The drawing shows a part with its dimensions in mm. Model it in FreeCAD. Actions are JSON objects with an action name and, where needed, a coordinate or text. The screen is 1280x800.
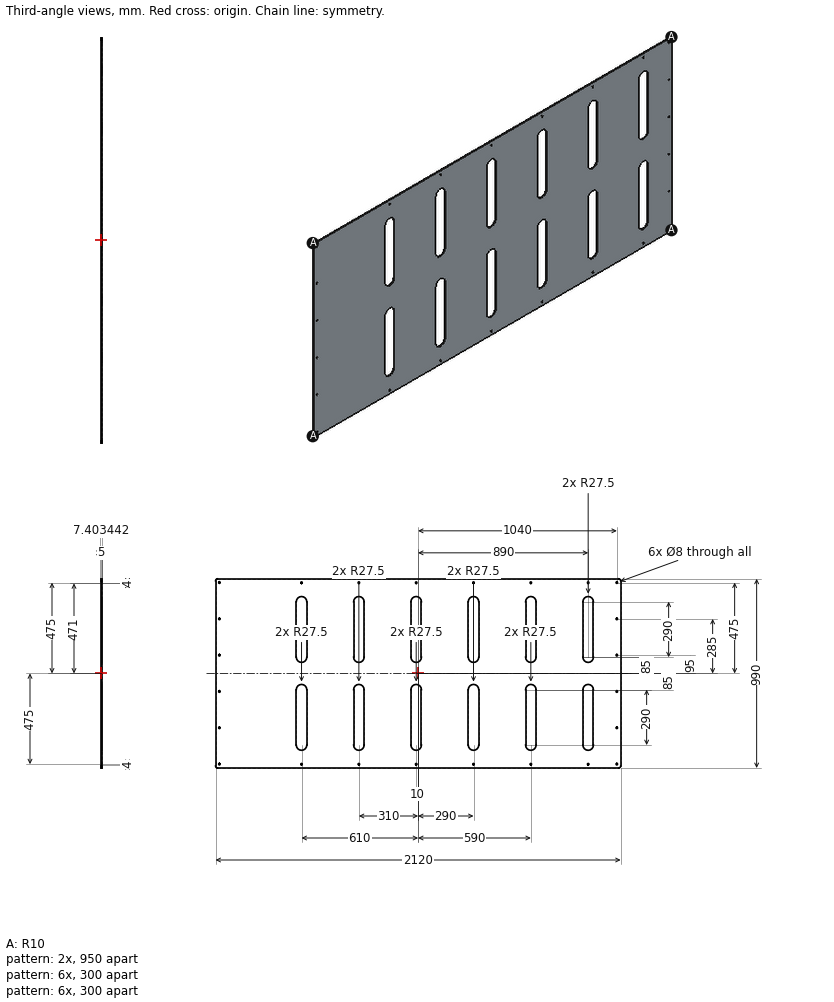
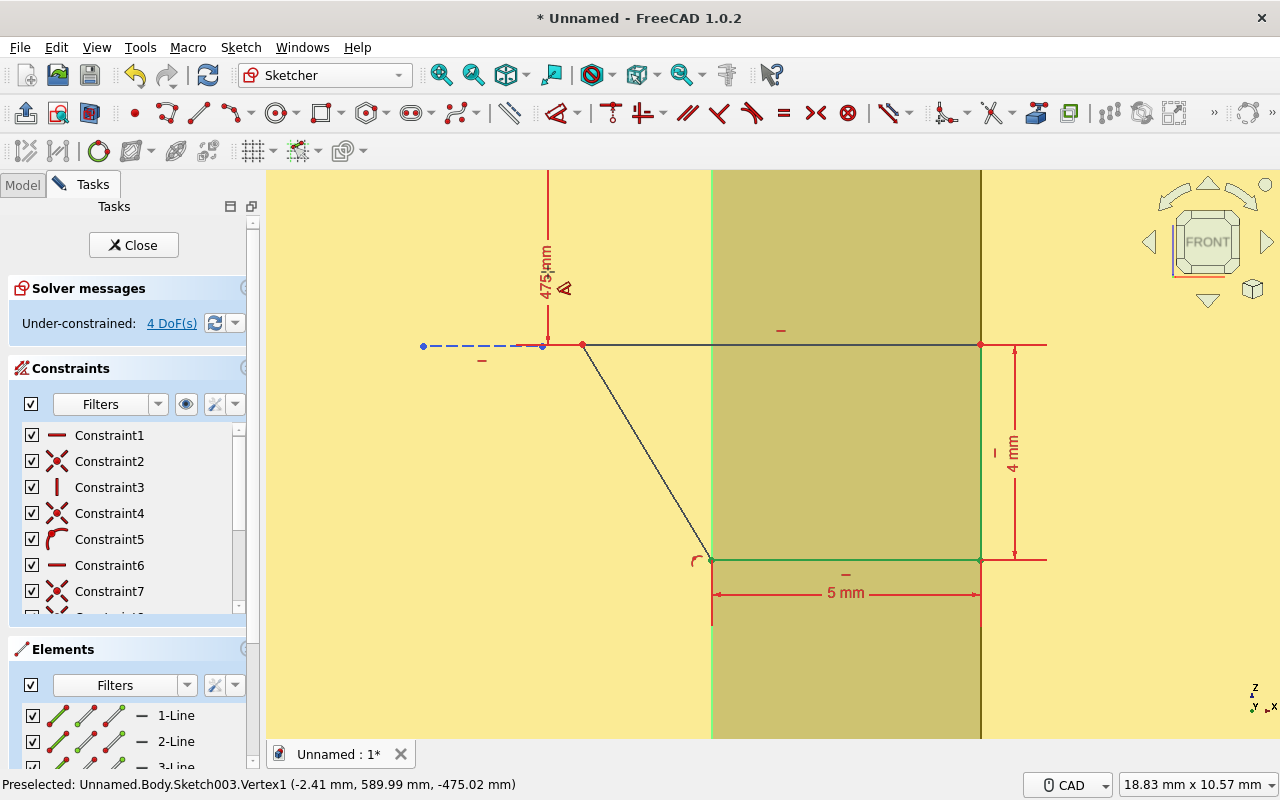
{"action": "left_click", "coordinate": [542, 346]}
{"action": "left_click", "coordinate": [508, 238]}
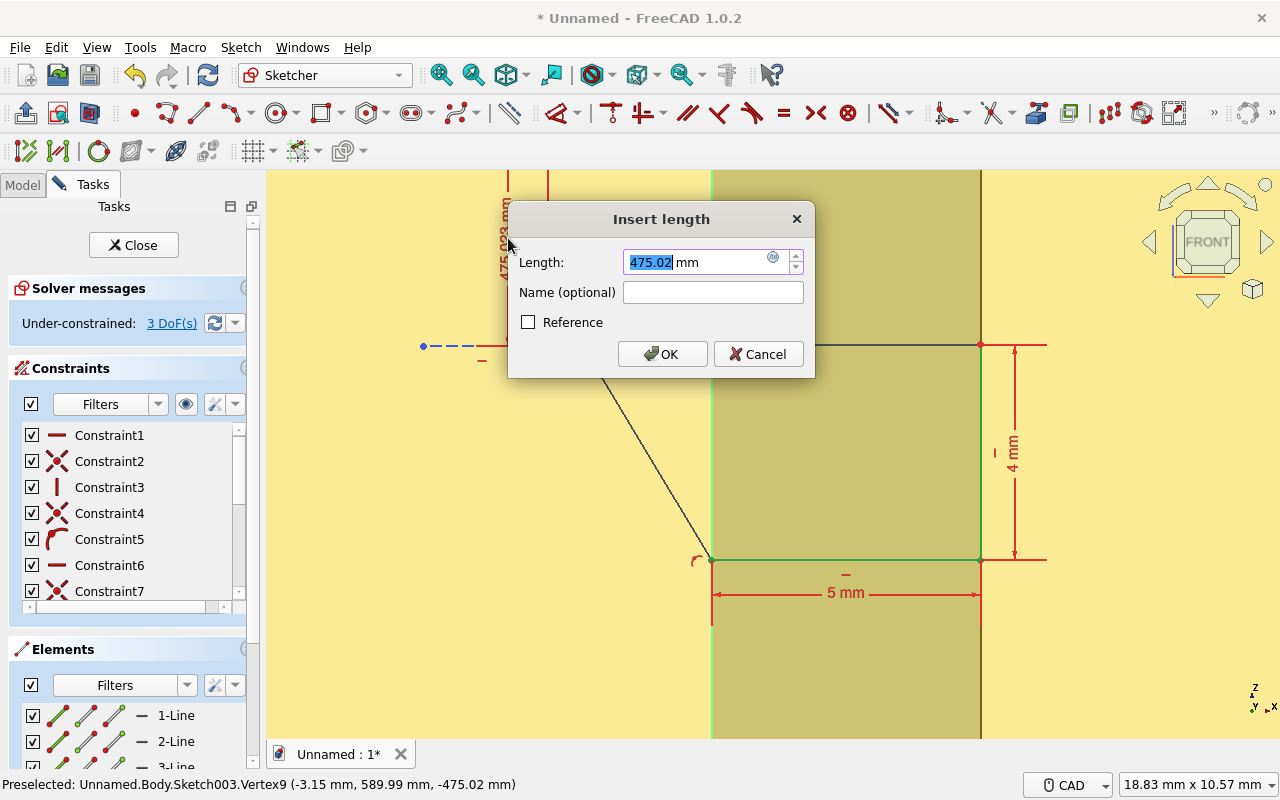
{"action": "type", "text": "475"}
{"action": "key", "text": "Return"}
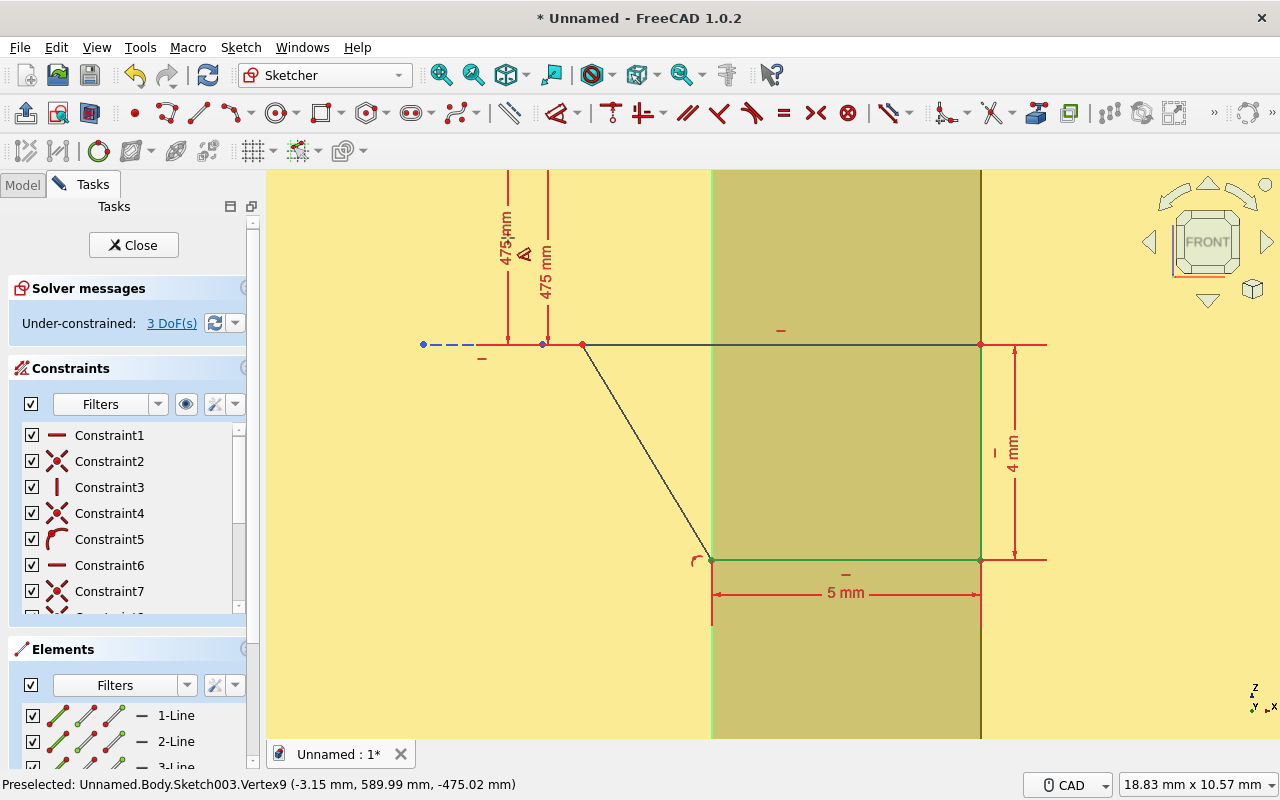
{"action": "scroll", "coordinate": [702, 345], "scroll_direction": "up", "scroll_amount": 2}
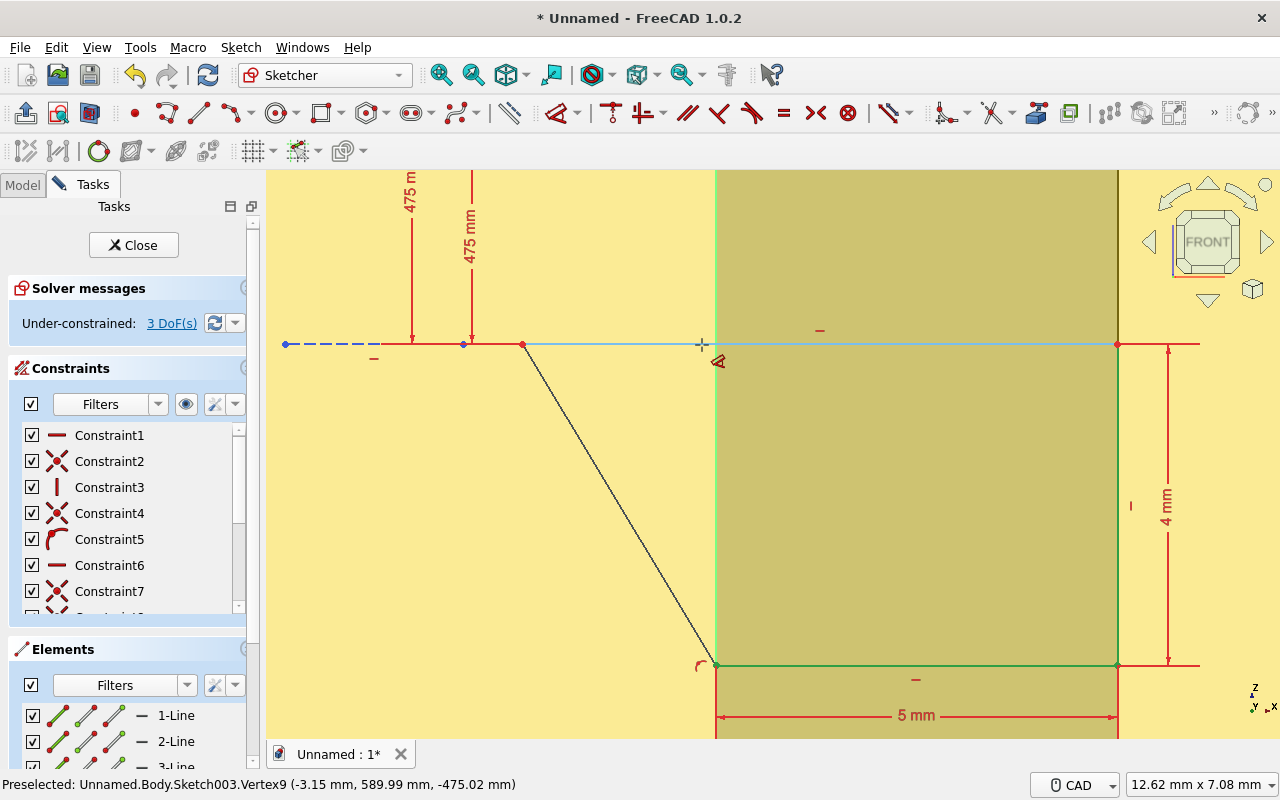
{"action": "left_click", "coordinate": [701, 344]}
{"action": "left_click", "coordinate": [819, 310]}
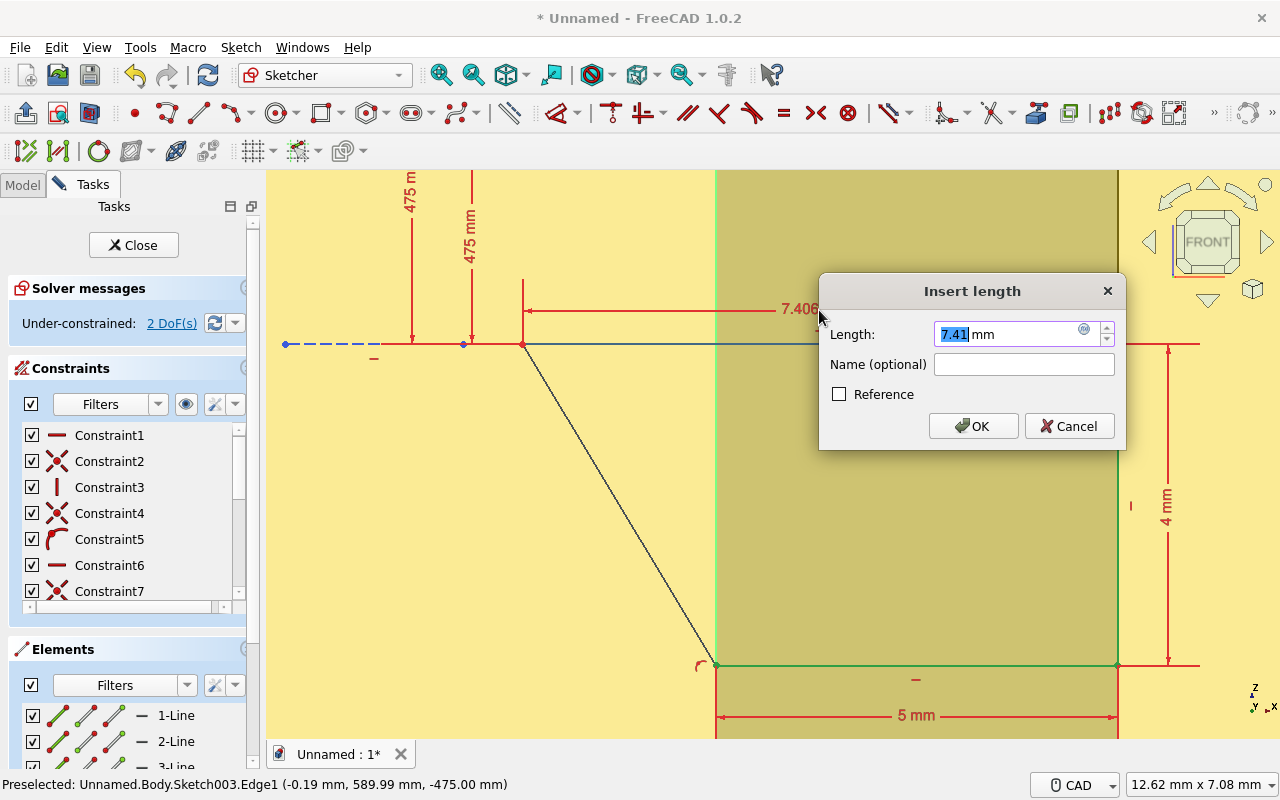
{"action": "type", "text": "7.403442"}
{"action": "key", "text": "Return"}
{"action": "key", "text": "Escape"}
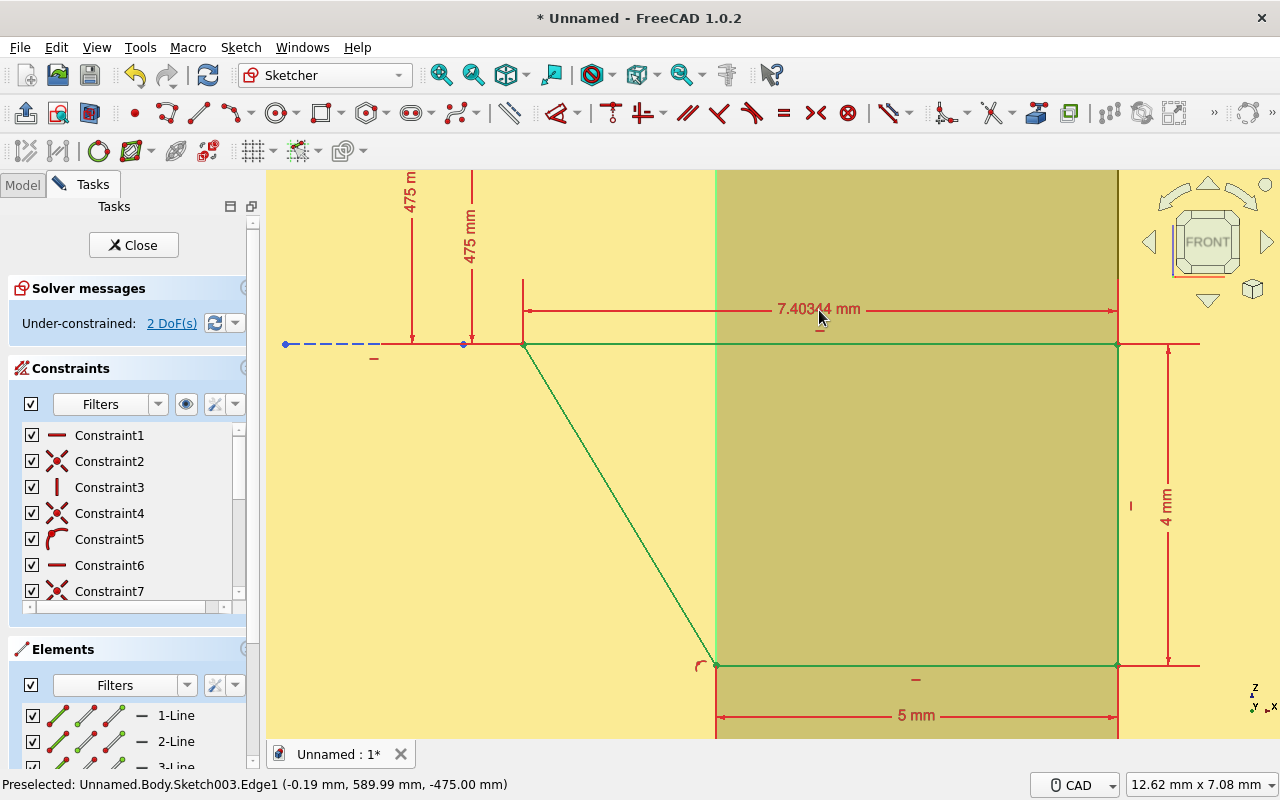
{"action": "left_click", "coordinate": [134, 245]}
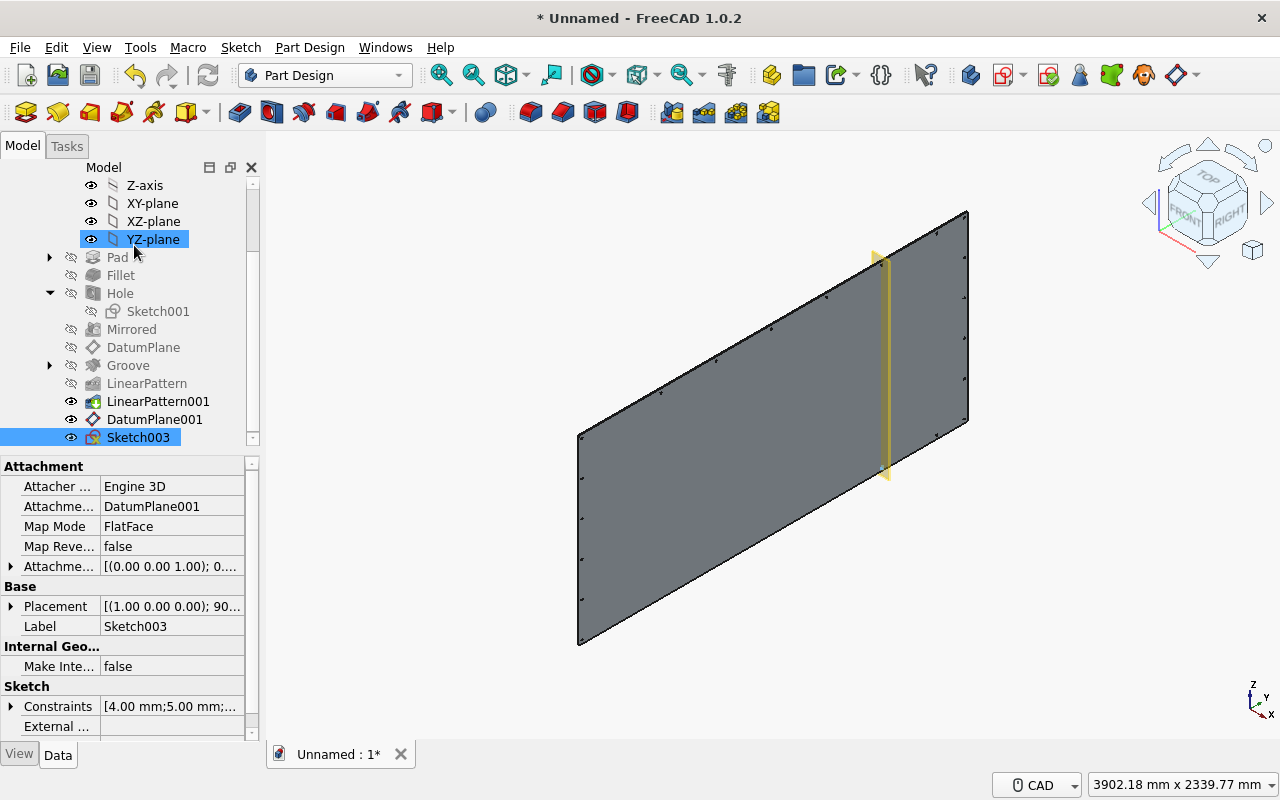
{"action": "left_click", "coordinate": [304, 112]}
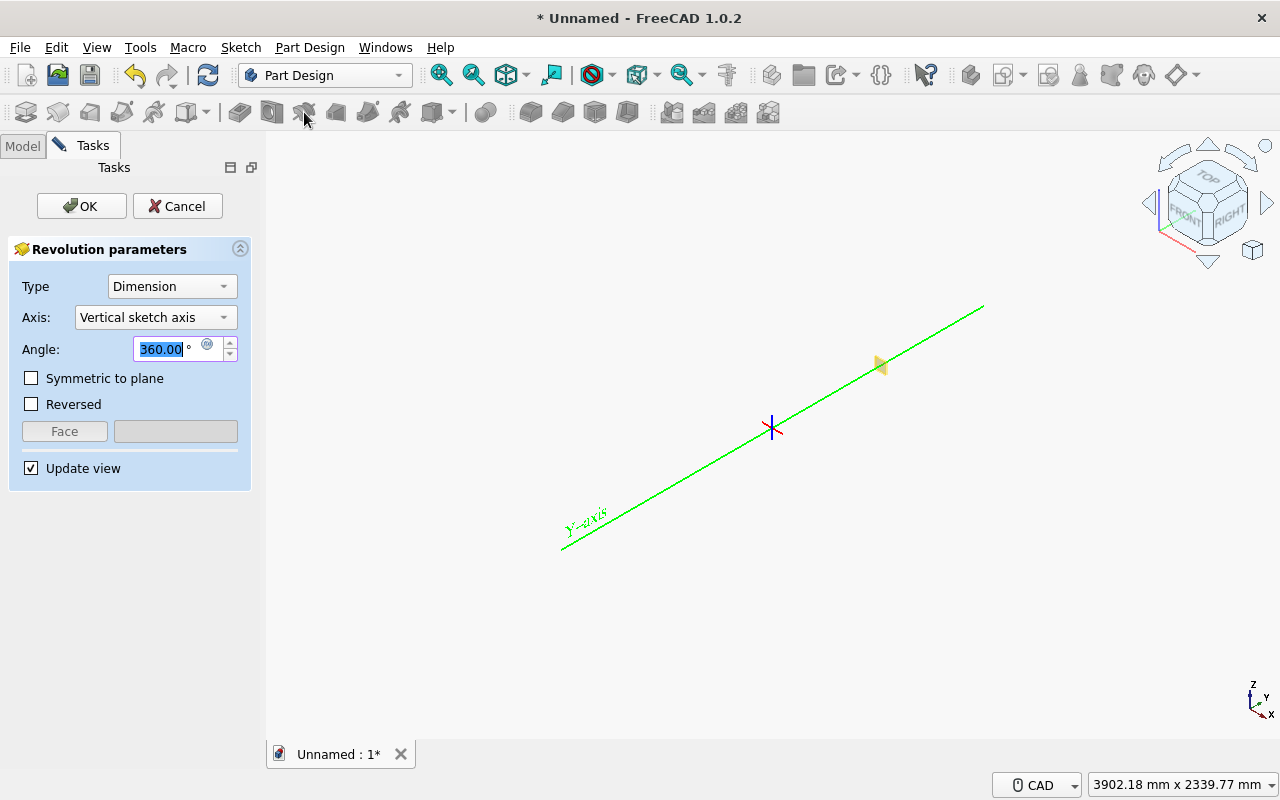
{"action": "left_click", "coordinate": [156, 318]}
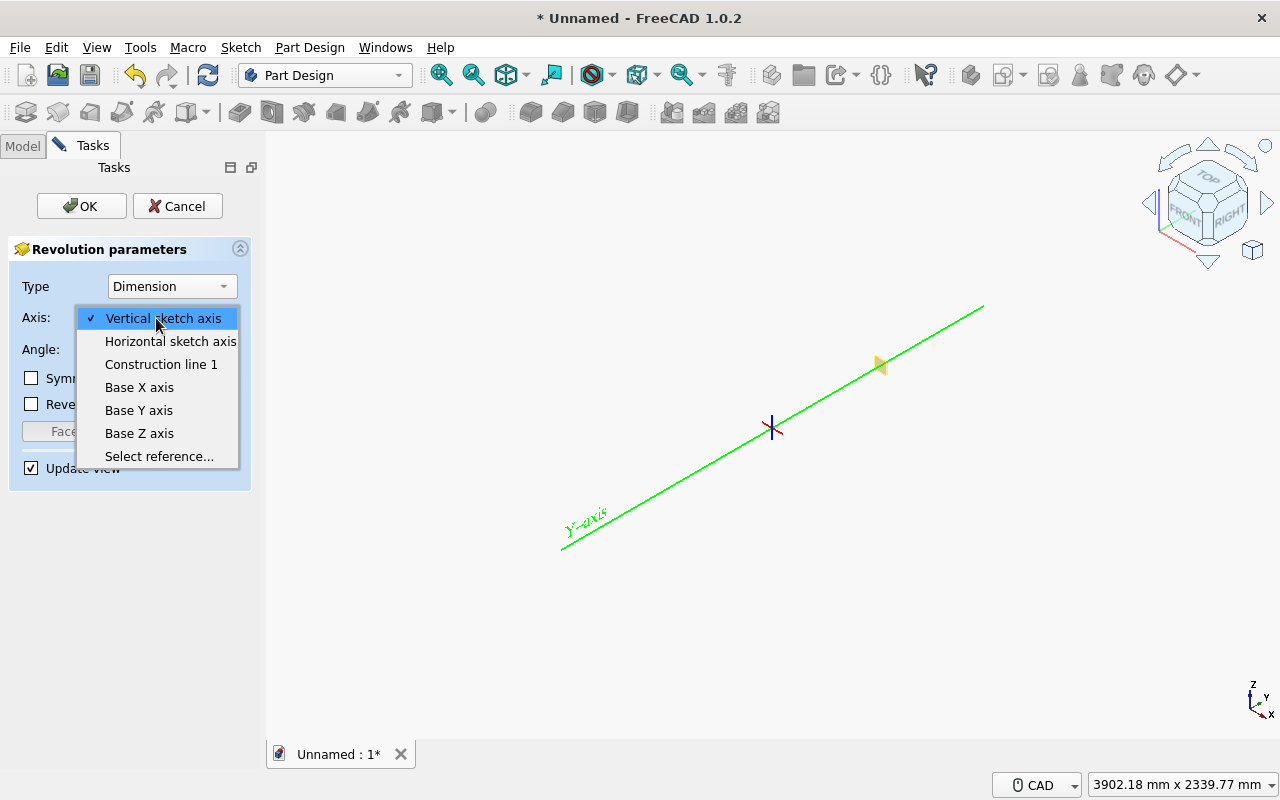
{"action": "left_click", "coordinate": [156, 364]}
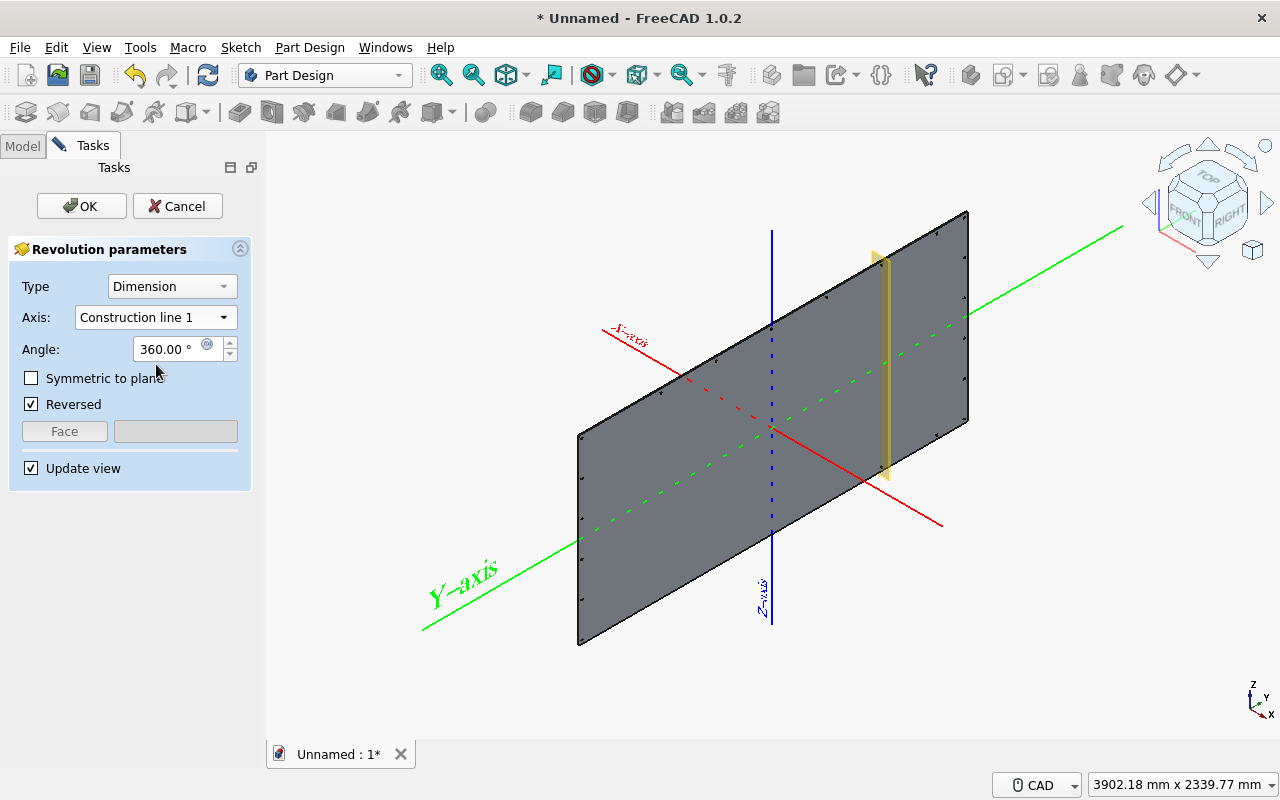
{"action": "left_click", "coordinate": [82, 206]}